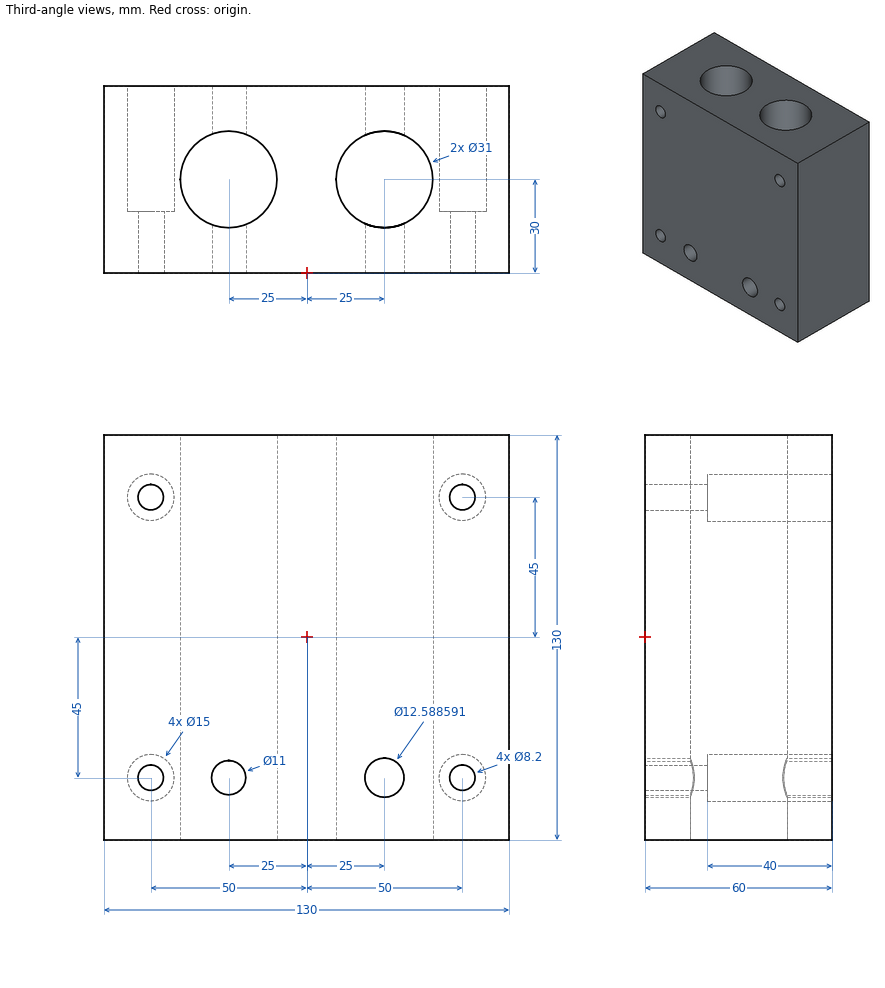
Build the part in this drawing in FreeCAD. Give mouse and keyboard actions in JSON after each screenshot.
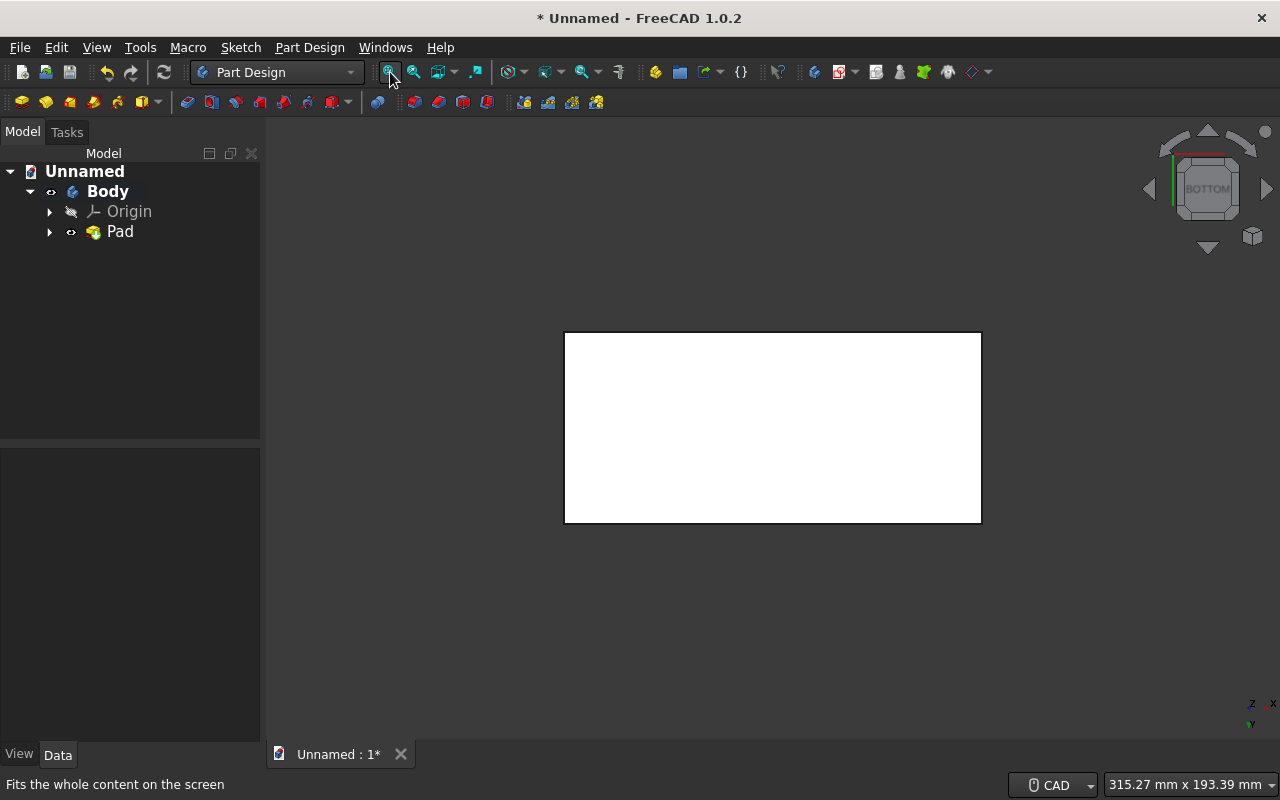
{"action": "key", "text": "v f"}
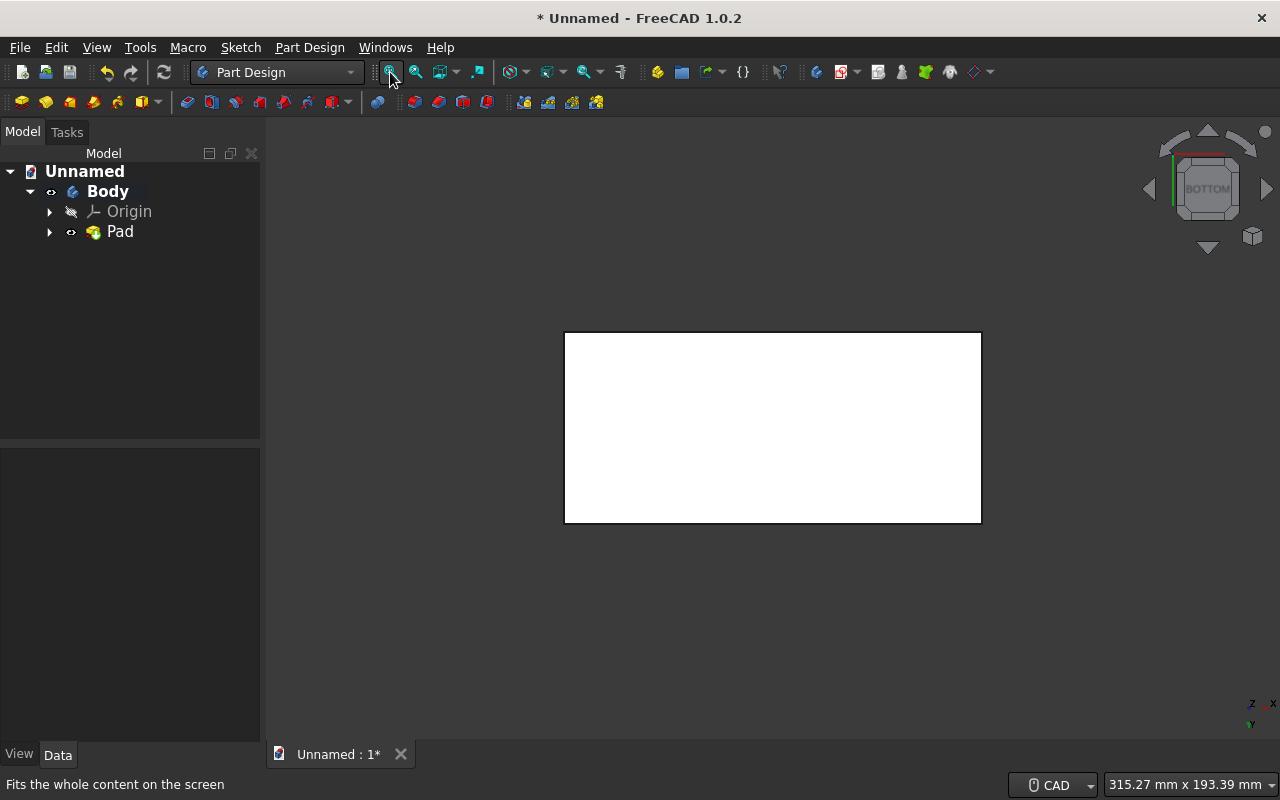
{"action": "left_click", "coordinate": [833, 427]}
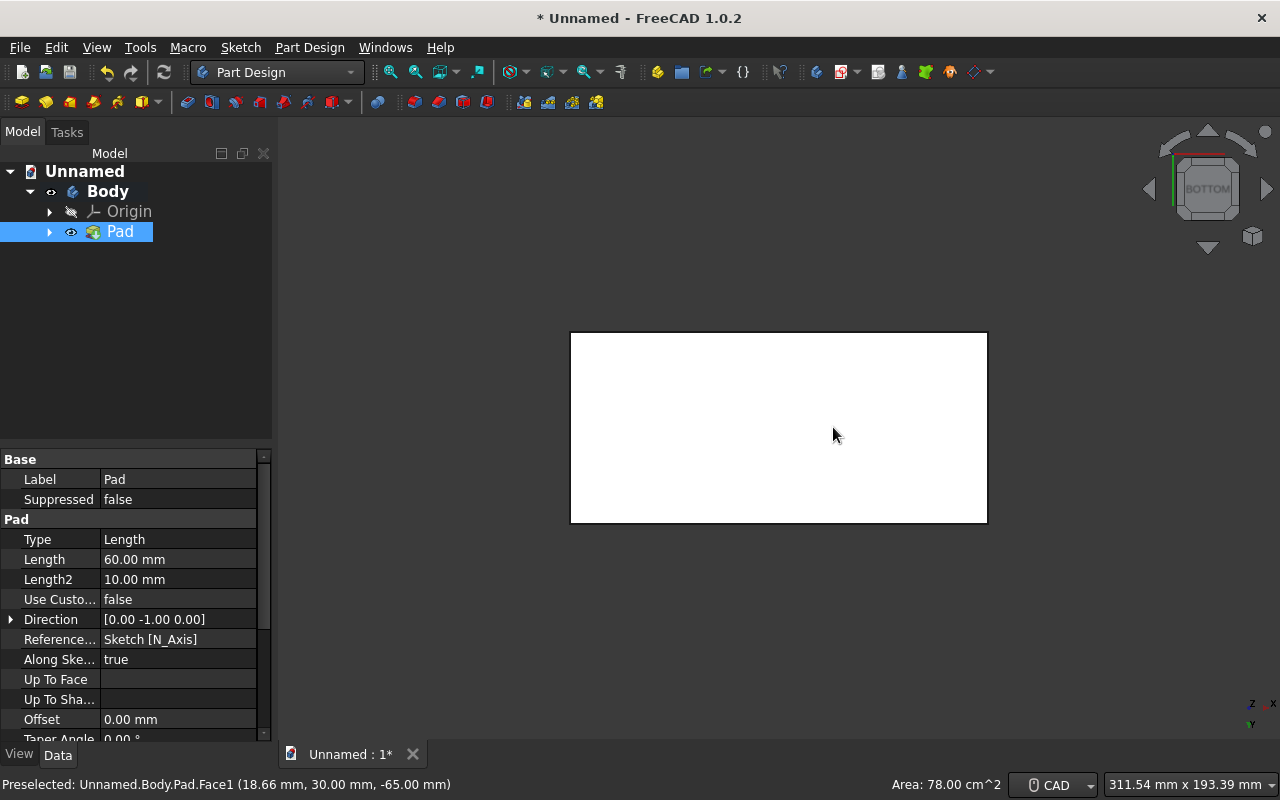
{"action": "left_click", "coordinate": [842, 72]}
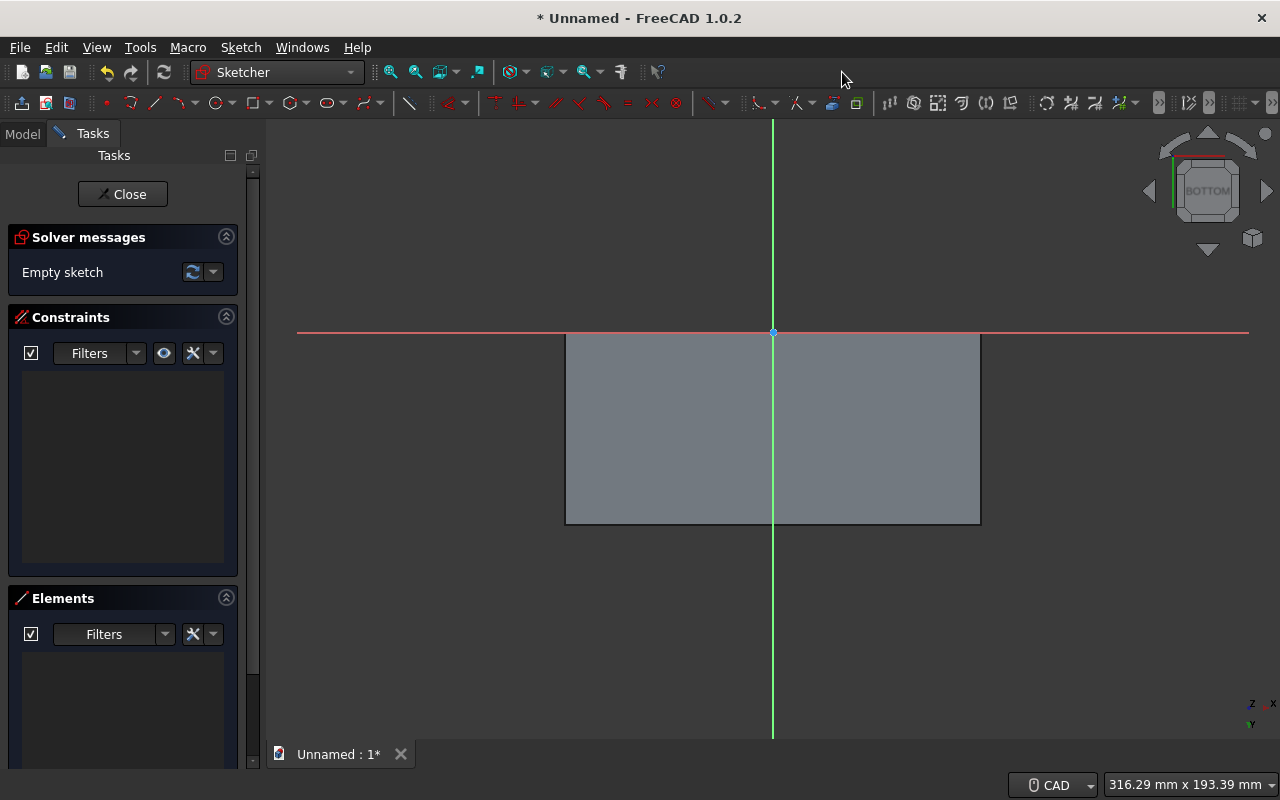
{"action": "scroll", "coordinate": [829, 387], "scroll_direction": "up", "scroll_amount": 4}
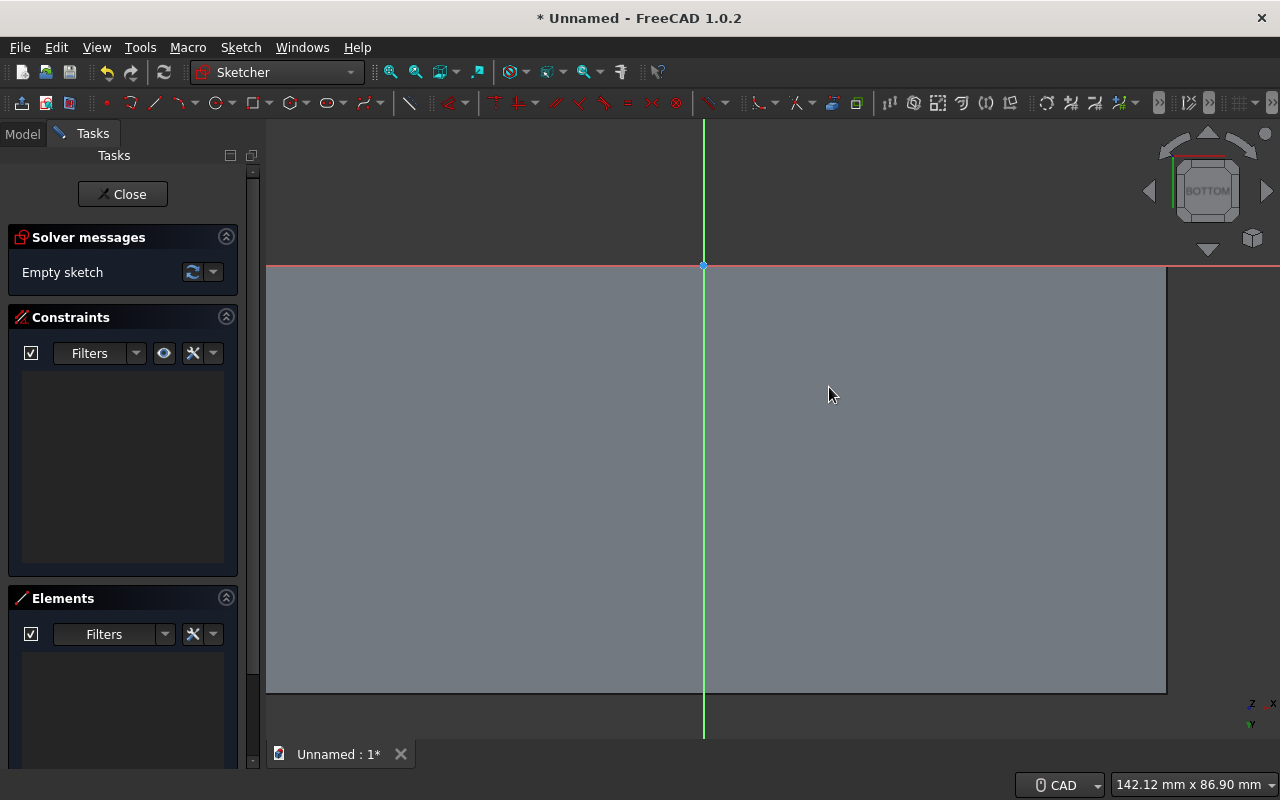
{"action": "left_click", "coordinate": [216, 104]}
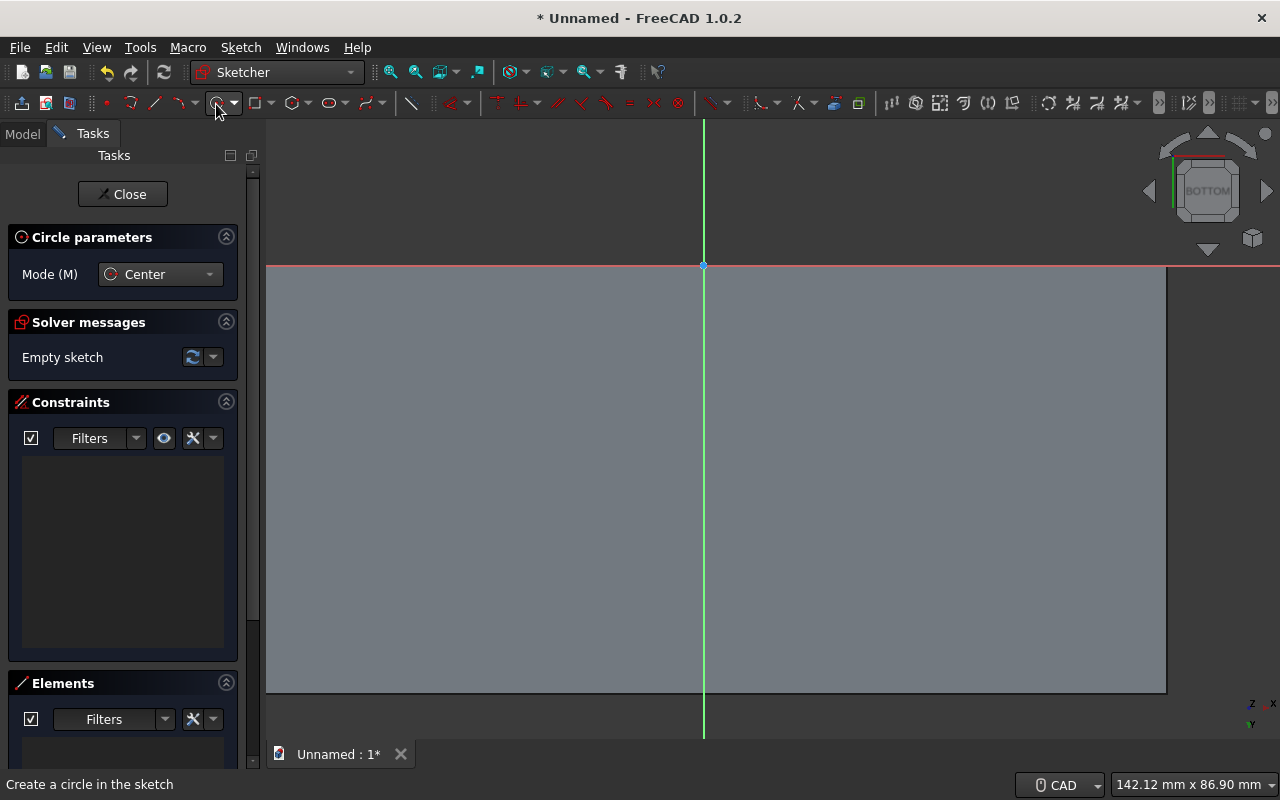
{"action": "left_click", "coordinate": [882, 480]}
{"action": "left_click", "coordinate": [960, 402]}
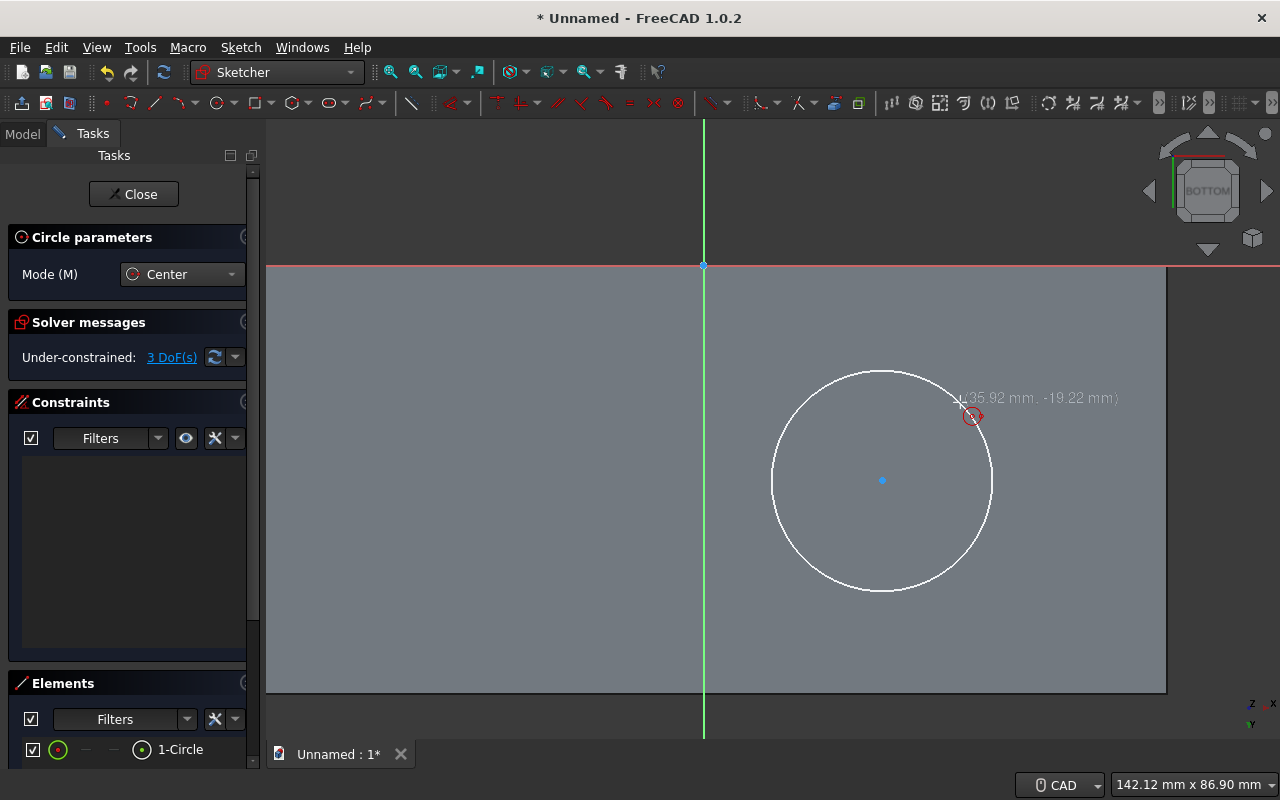
{"action": "left_click", "coordinate": [525, 480]}
{"action": "left_click", "coordinate": [604, 402]}
{"action": "key", "text": "Escape"}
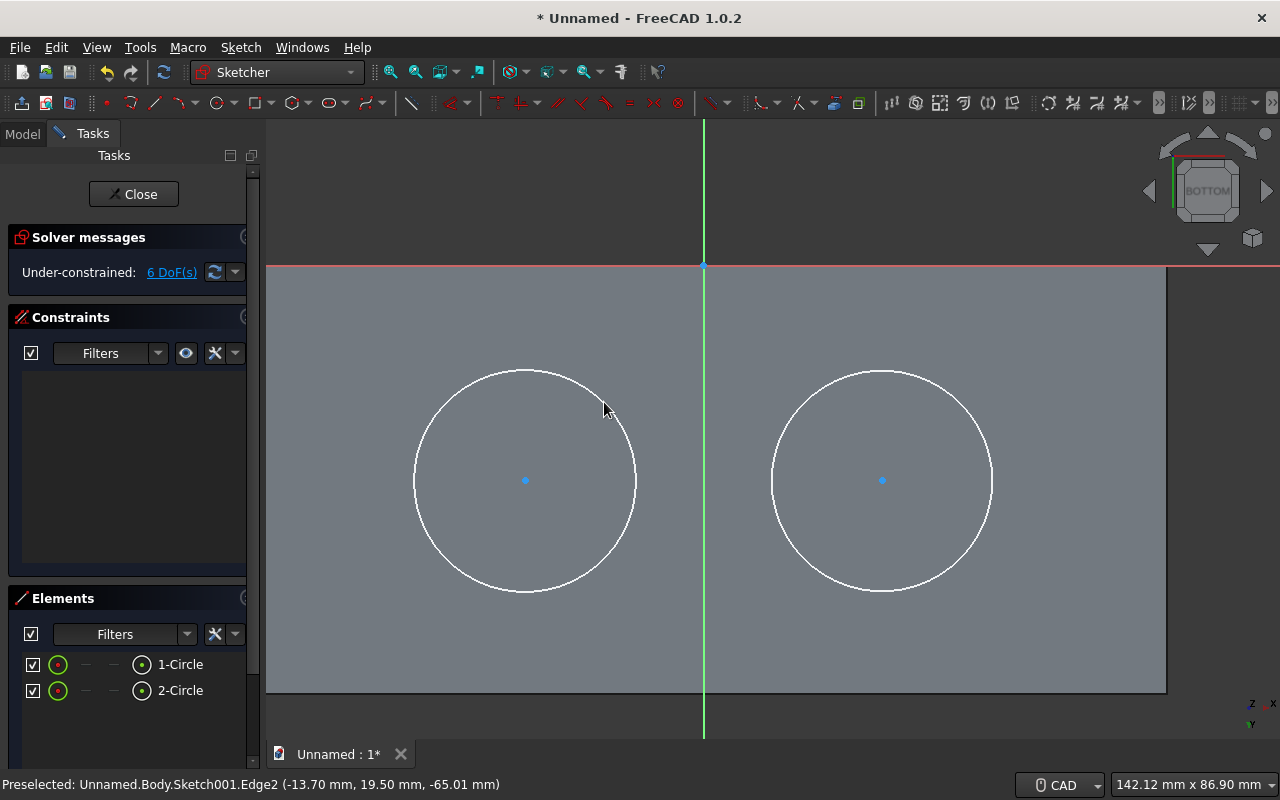
{"action": "left_click", "coordinate": [960, 403]}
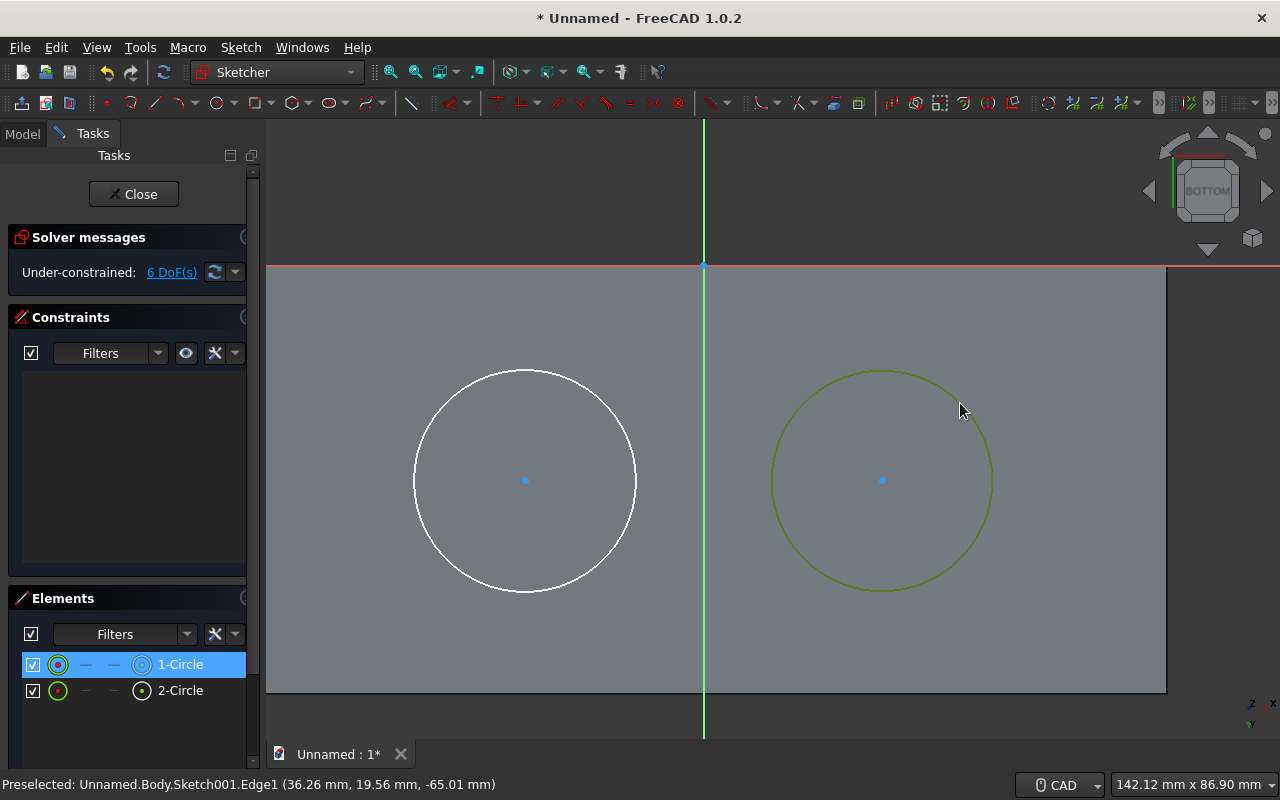
{"action": "left_click", "coordinate": [603, 402]}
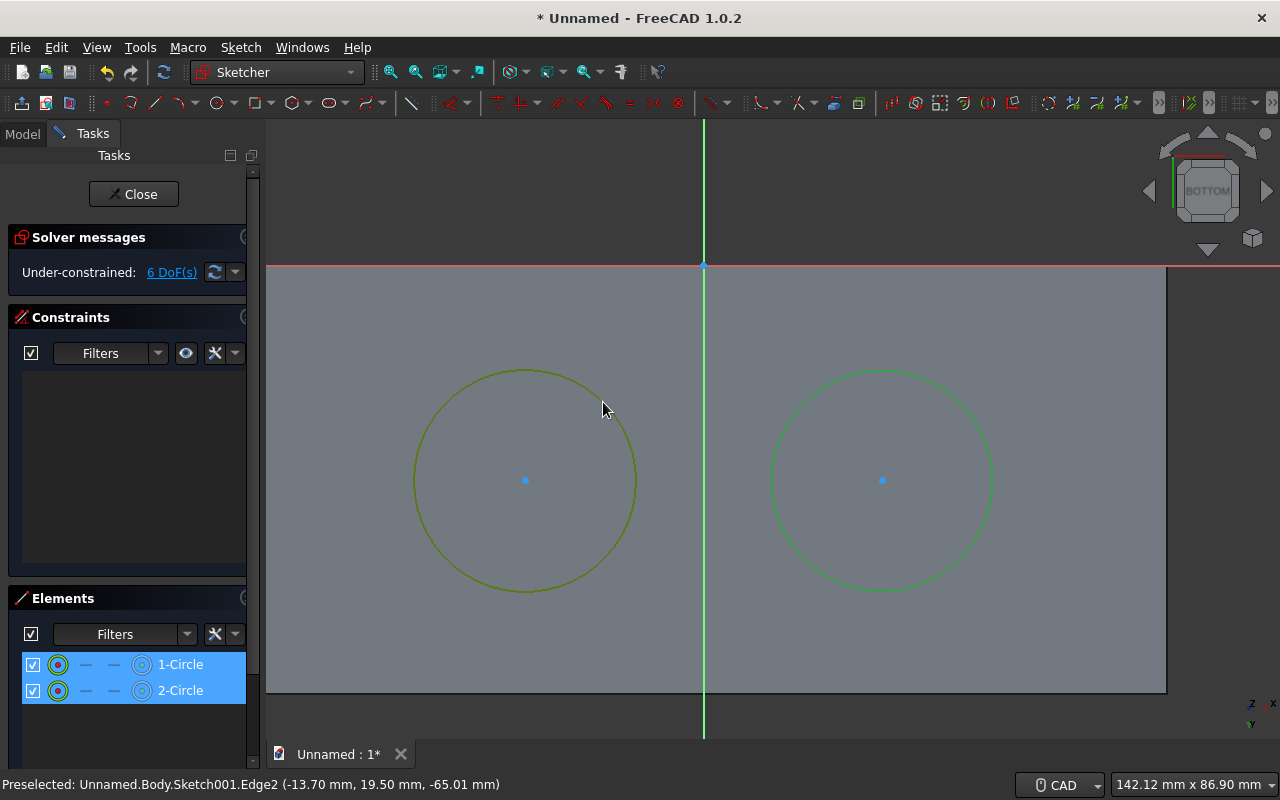
{"action": "left_click", "coordinate": [630, 104]}